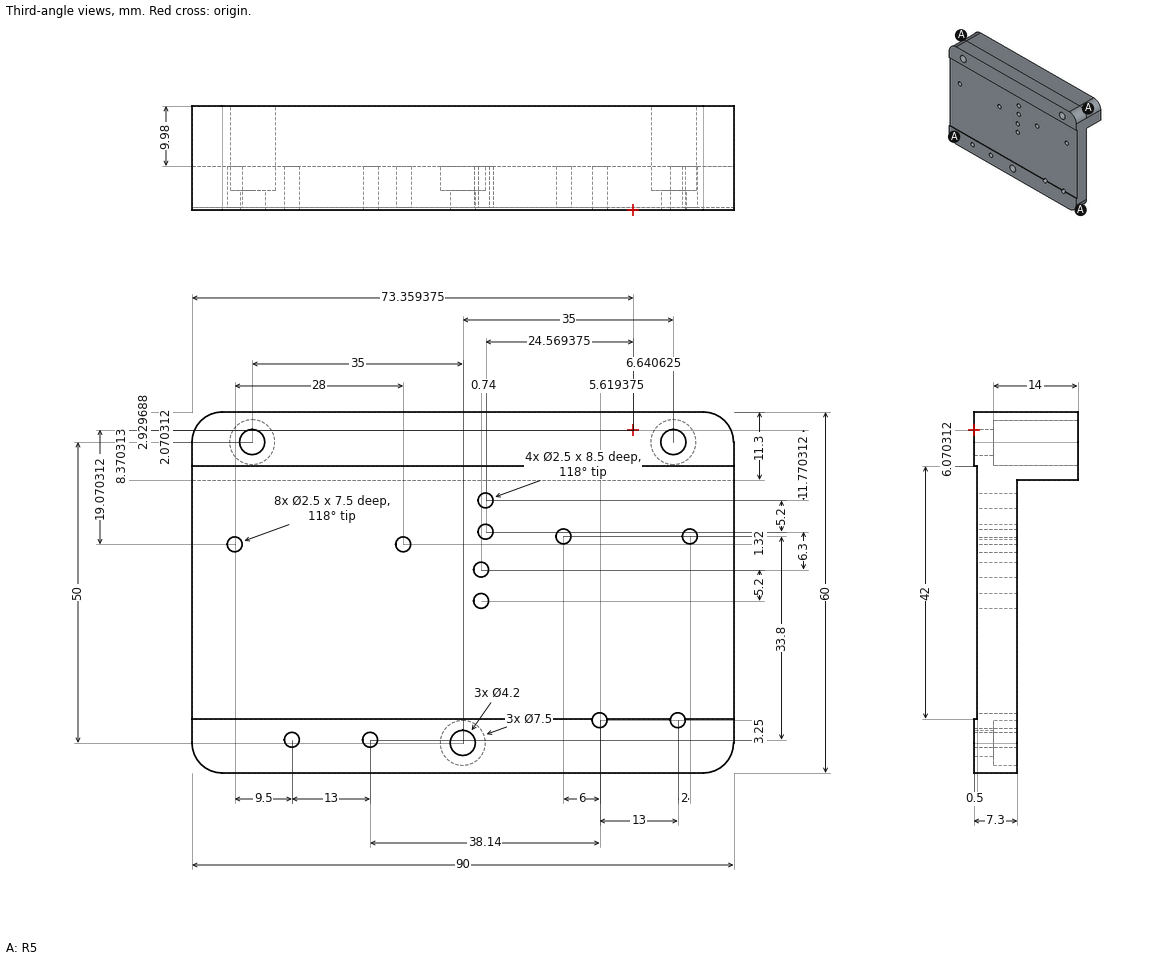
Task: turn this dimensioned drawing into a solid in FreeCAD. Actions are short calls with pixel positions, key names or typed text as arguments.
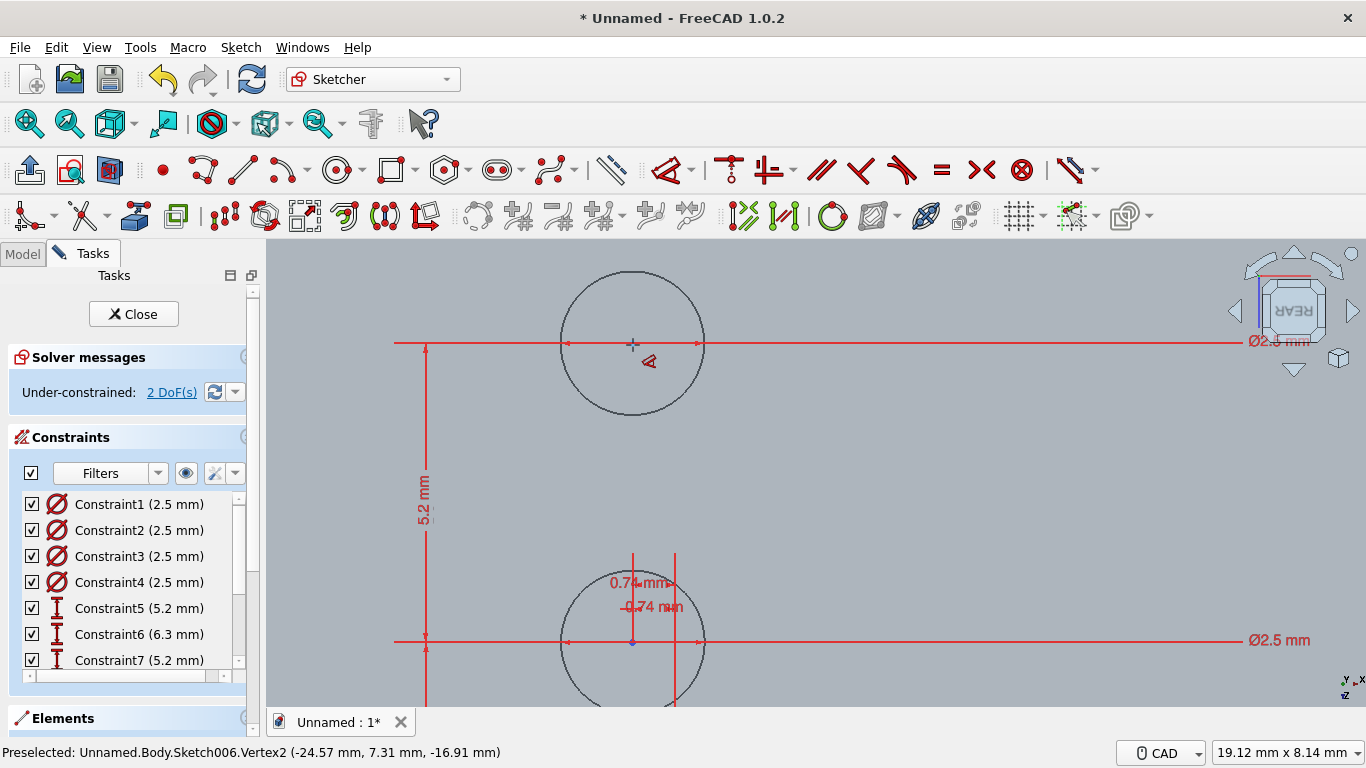
click(632, 343)
click(654, 309)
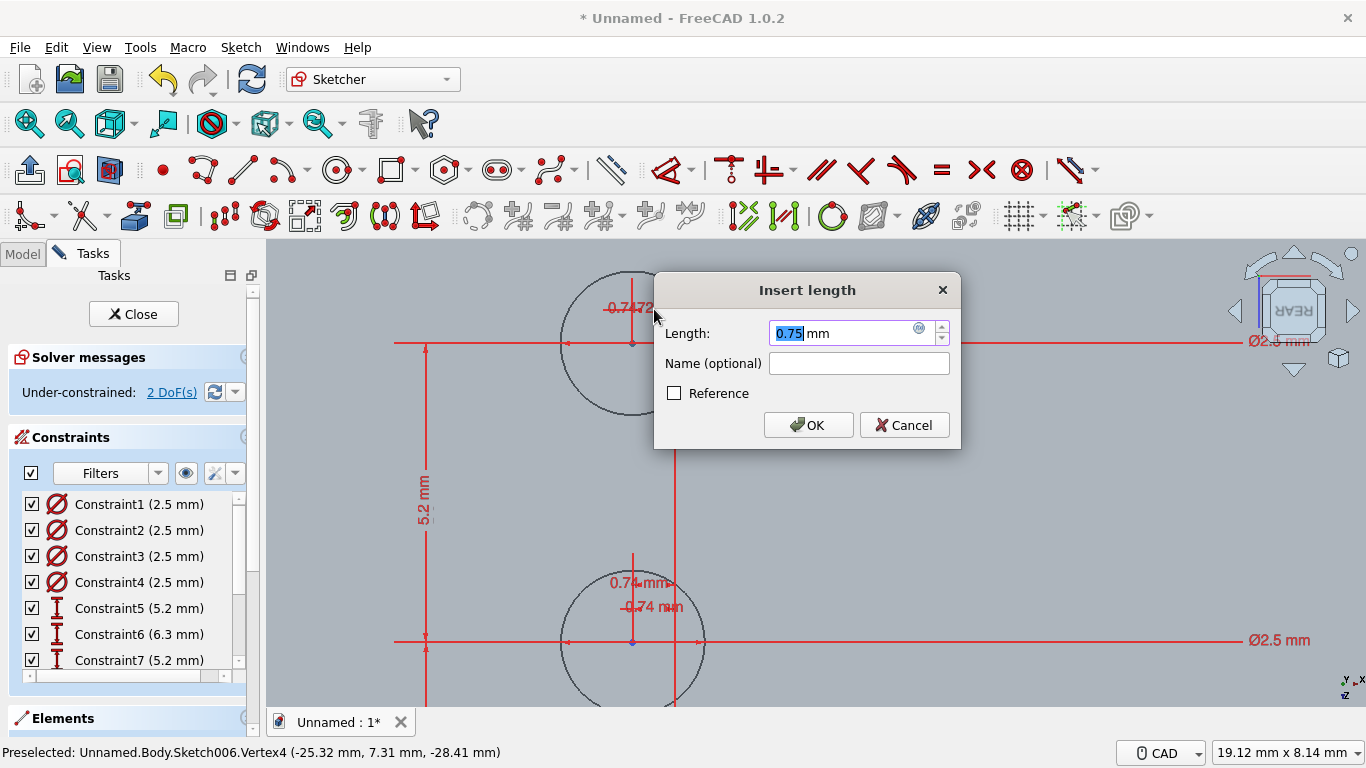
text(0.74)
key(Return)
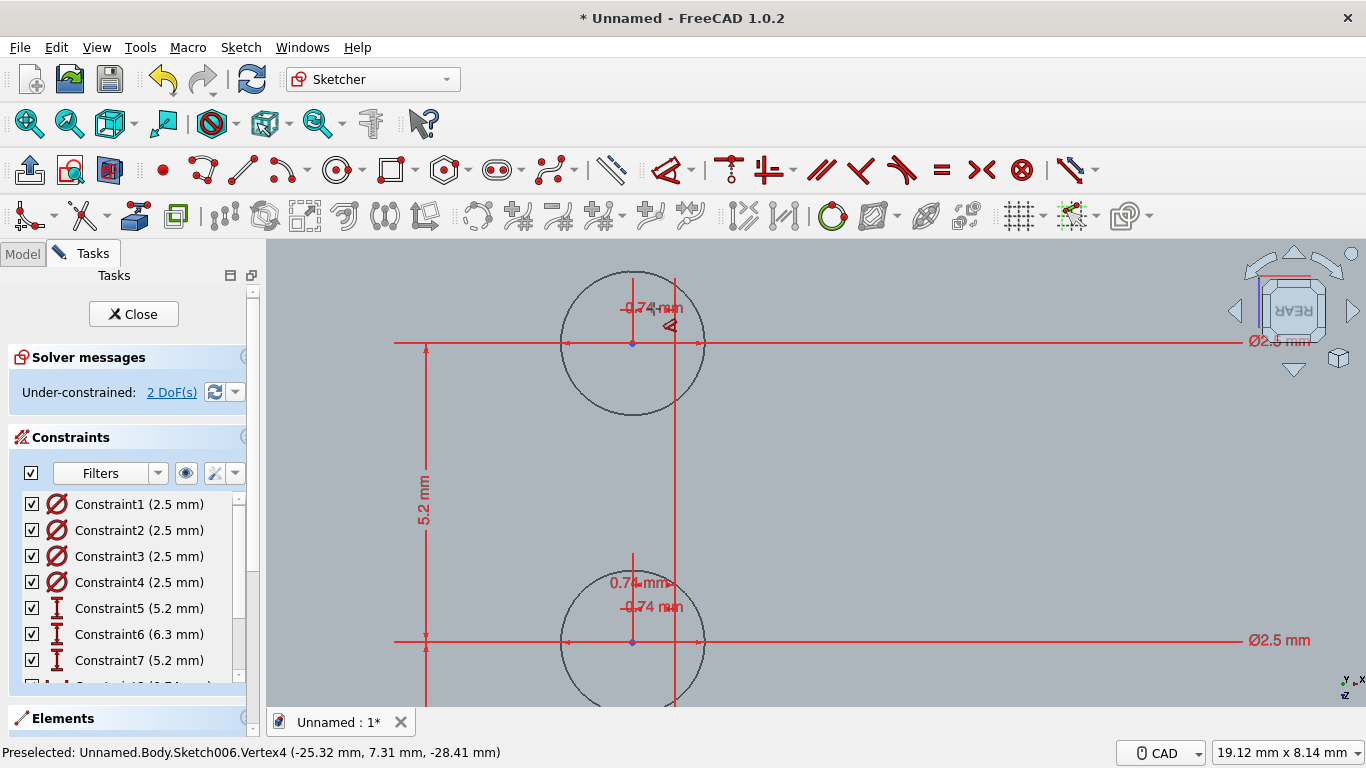
scroll(633, 344, down, 9)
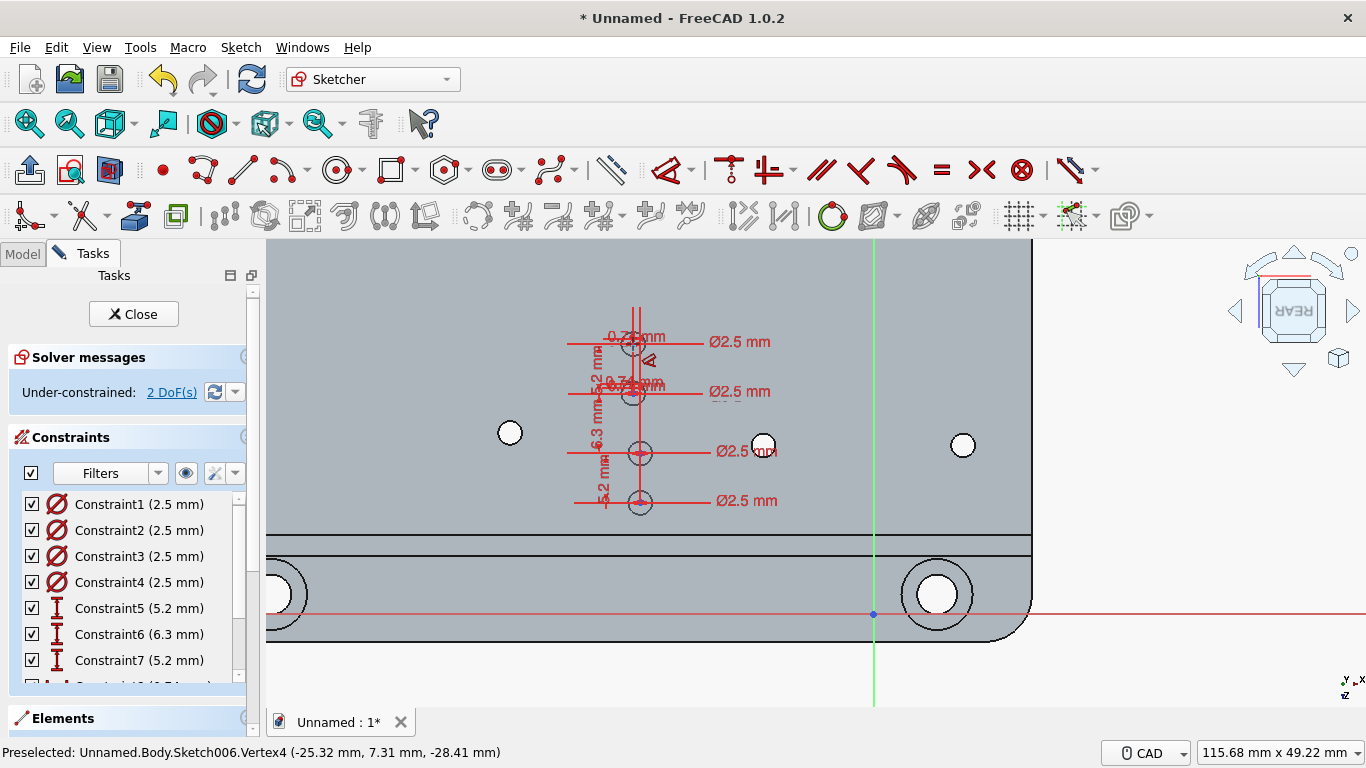
click(640, 503)
click(757, 648)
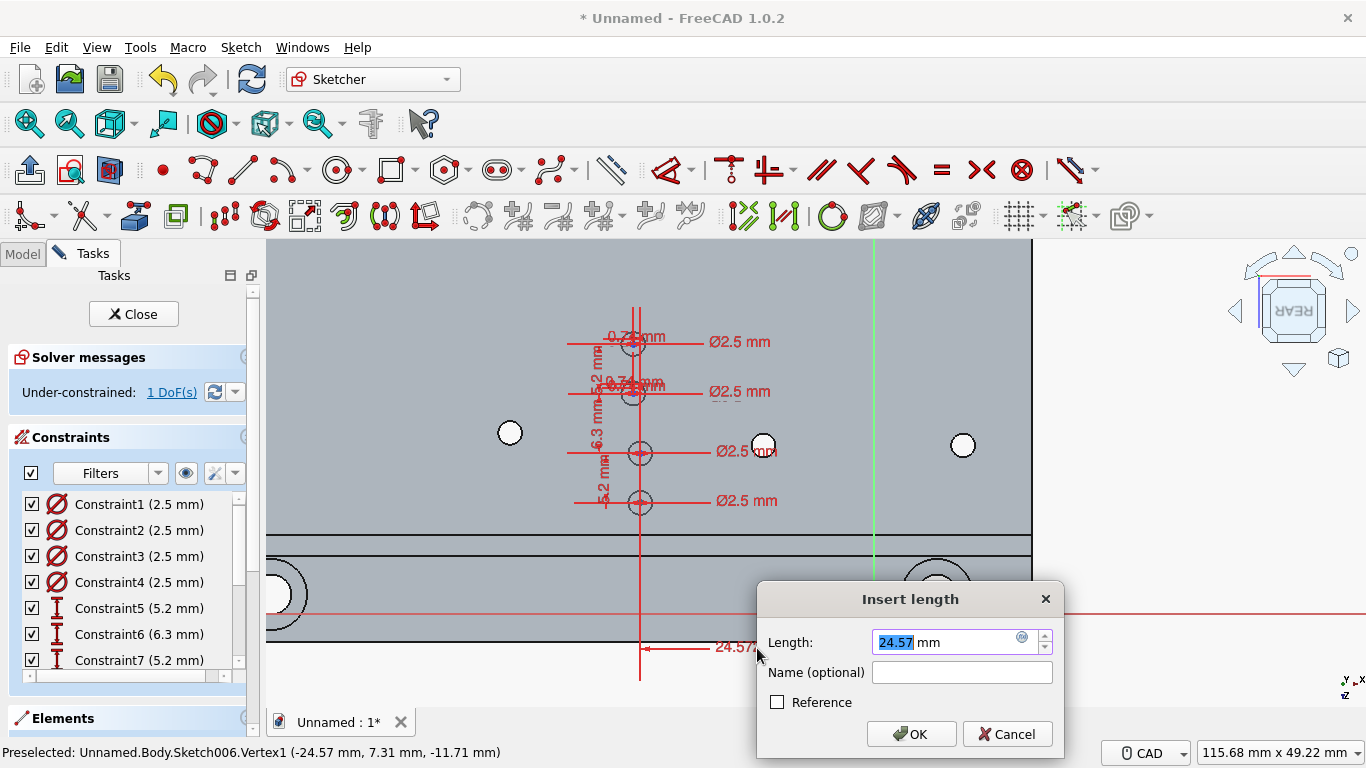
text(24.569375)
key(Return)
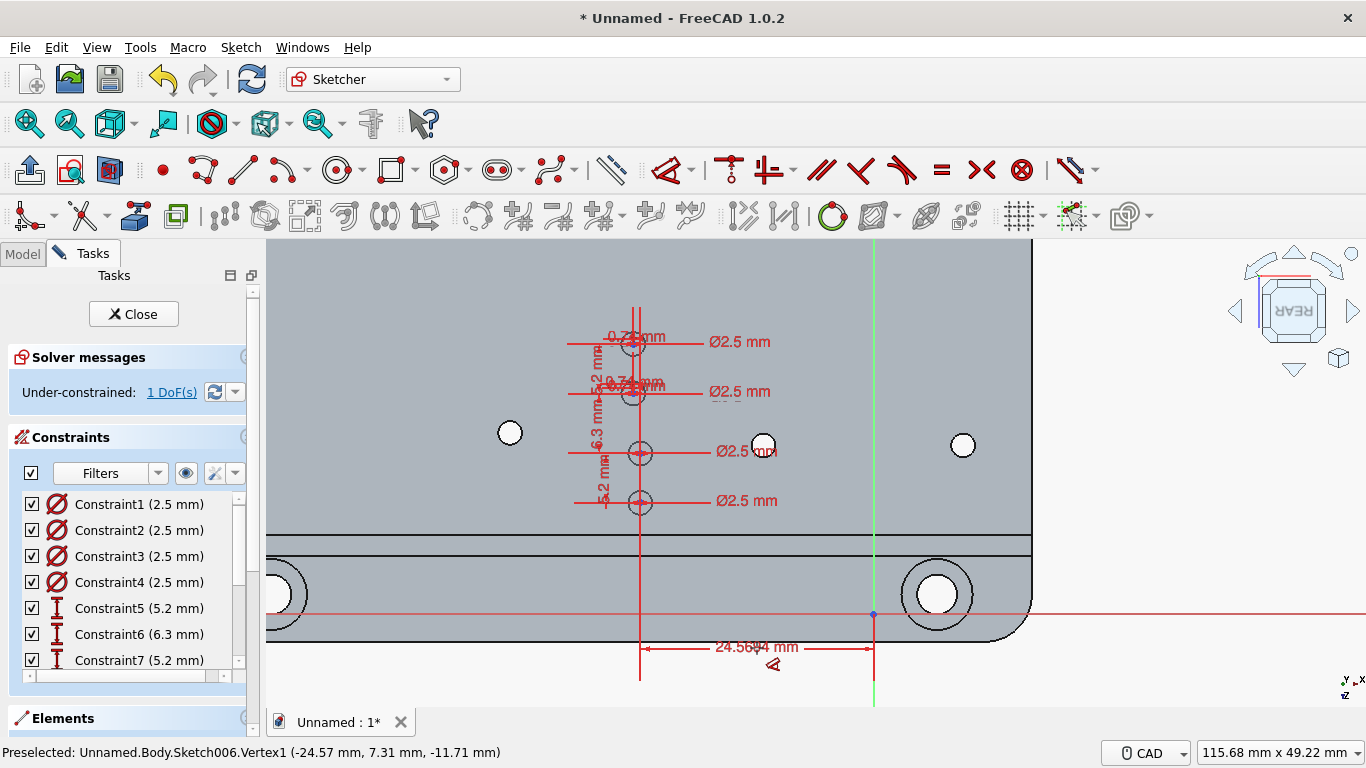
click(640, 503)
click(908, 559)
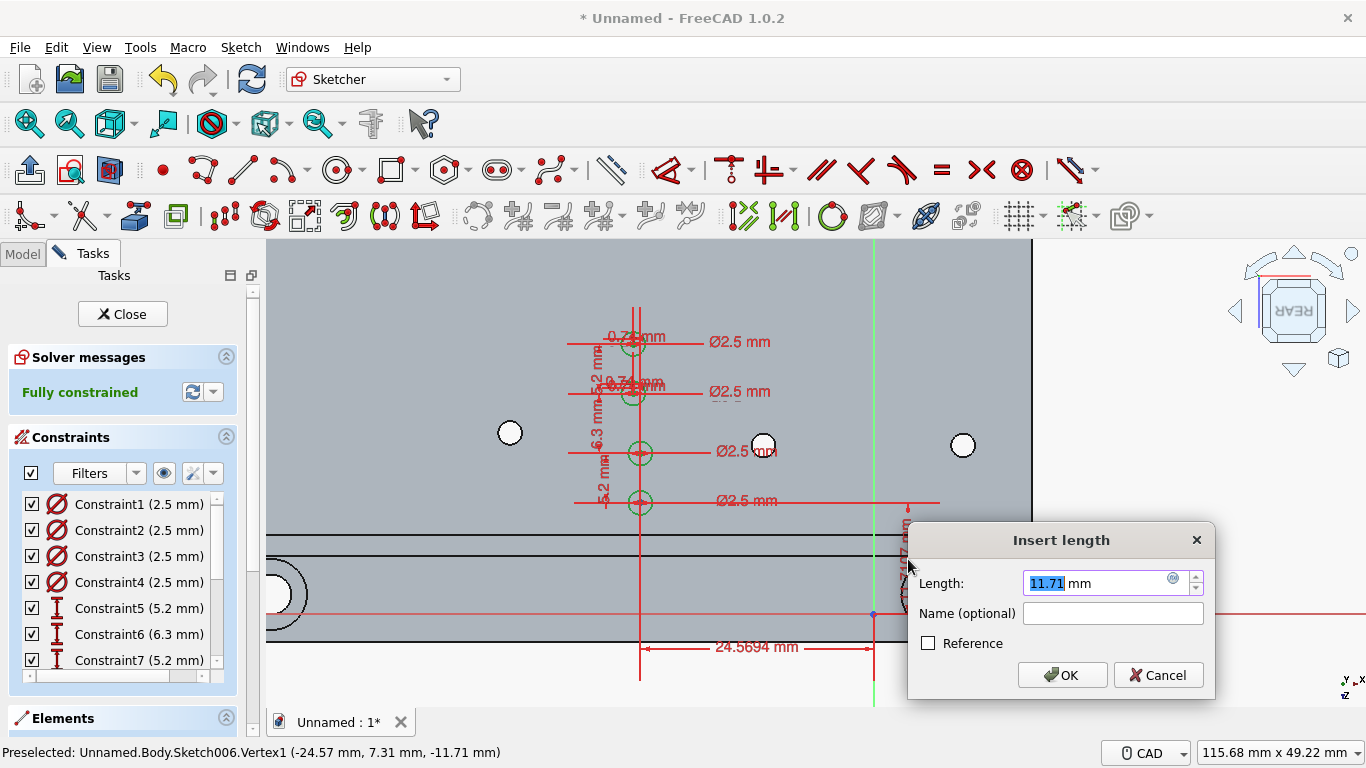
text(11.770312)
key(Return)
key(Escape)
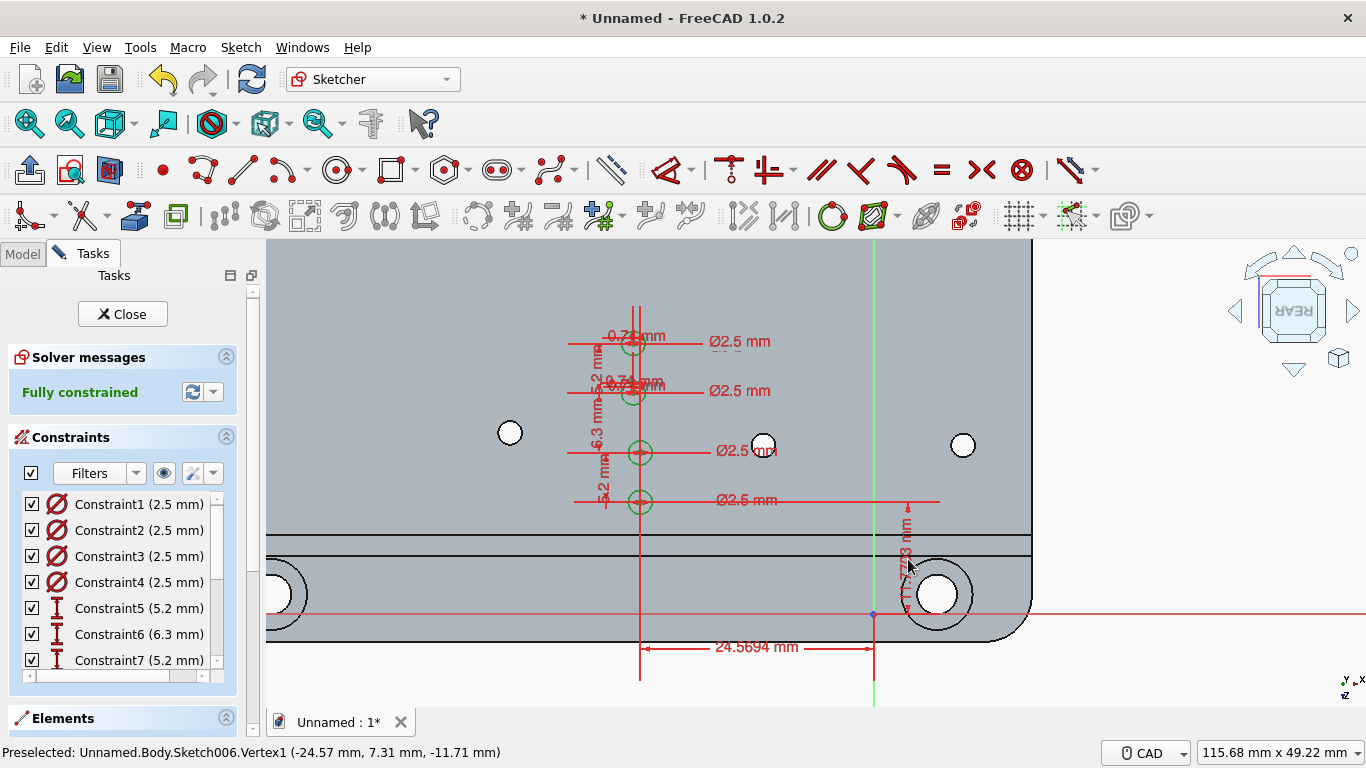
click(123, 314)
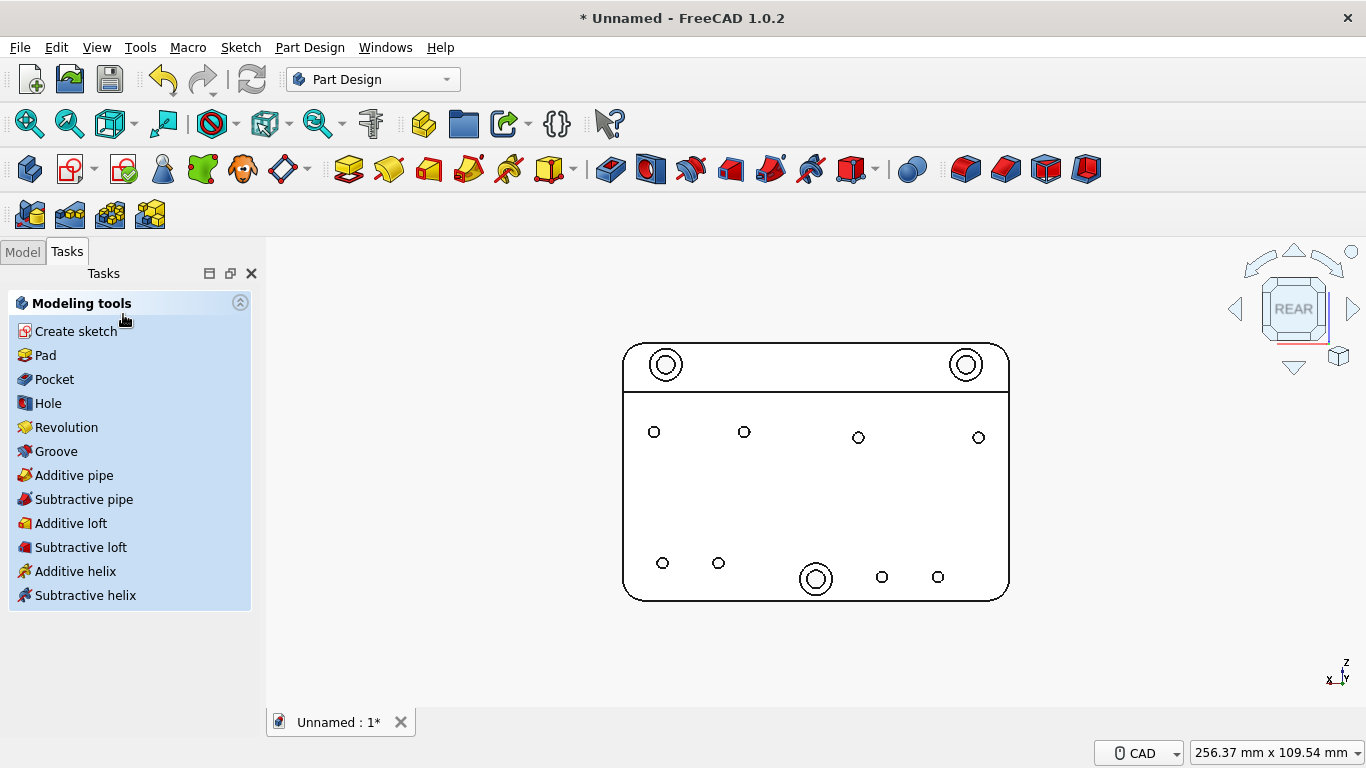
click(652, 170)